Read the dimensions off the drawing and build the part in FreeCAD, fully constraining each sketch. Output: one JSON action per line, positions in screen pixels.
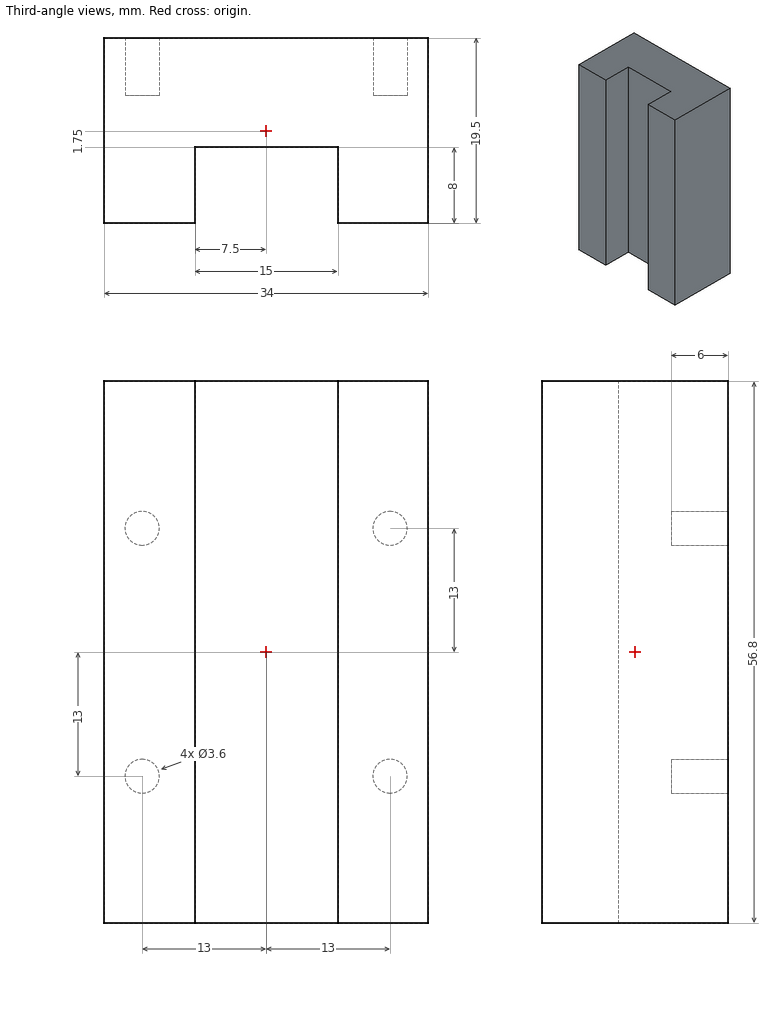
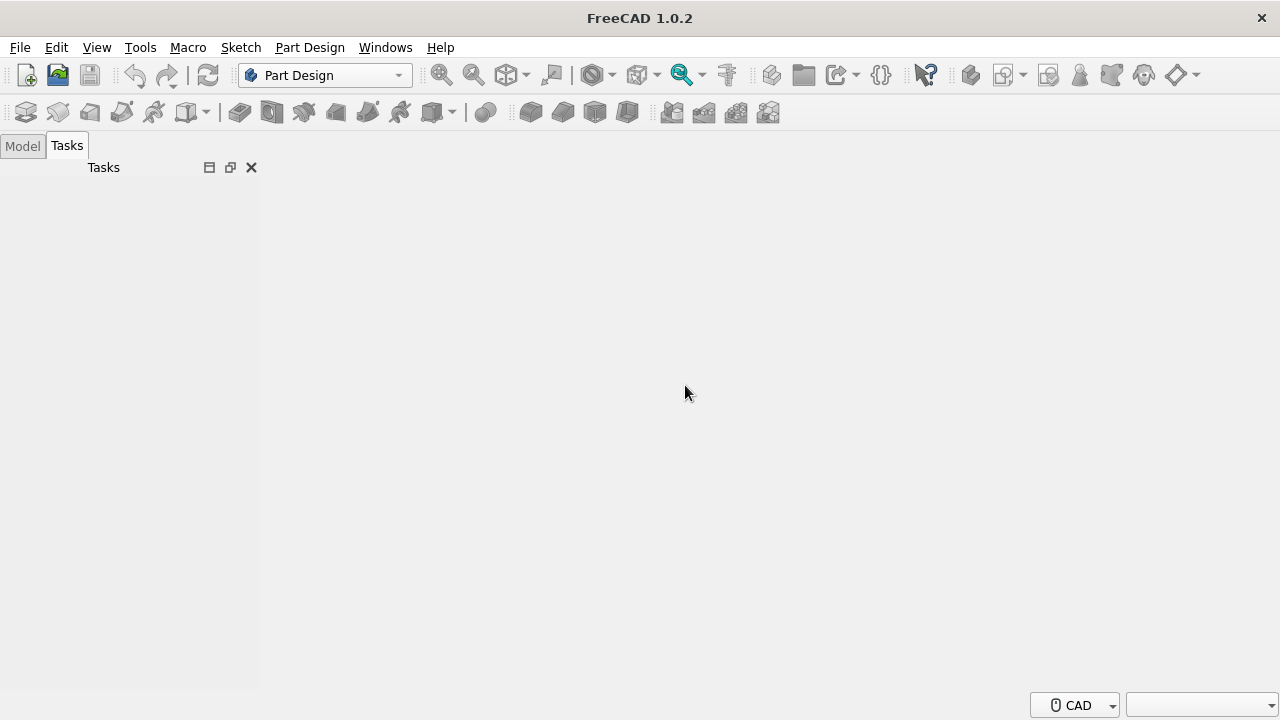
{"action": "left_click", "coordinate": [26, 76]}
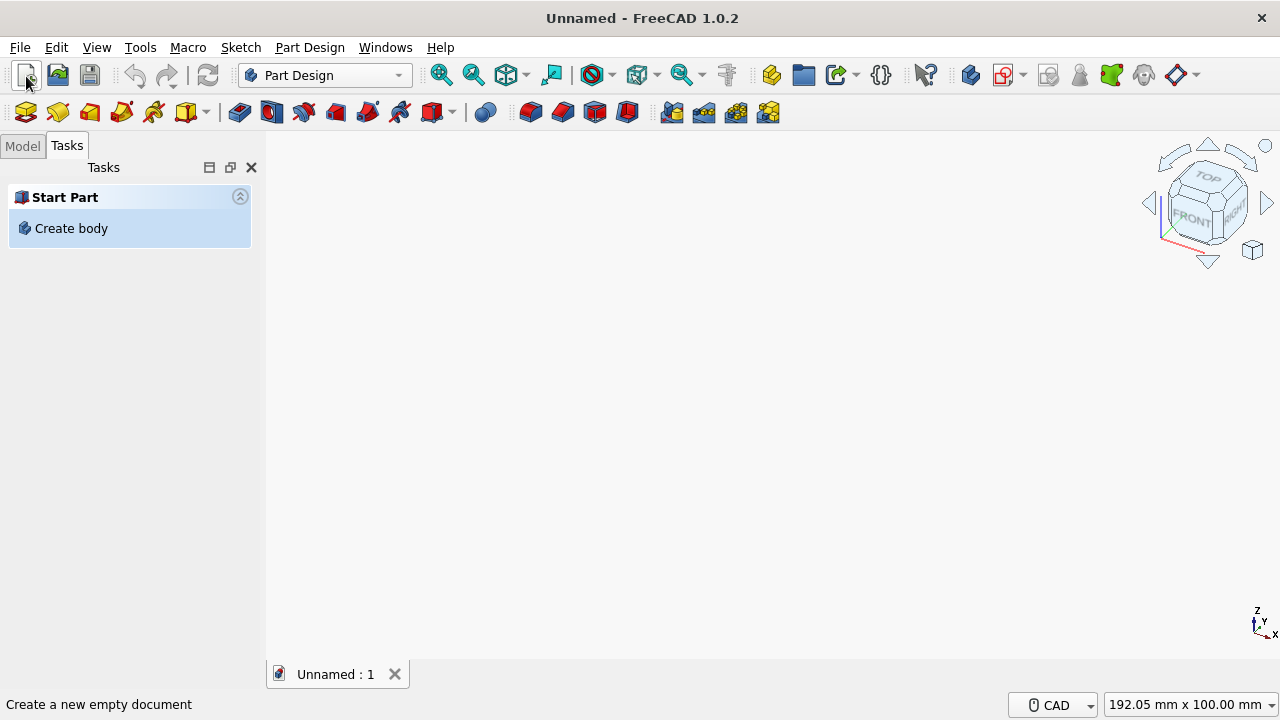
{"action": "left_click", "coordinate": [1004, 76]}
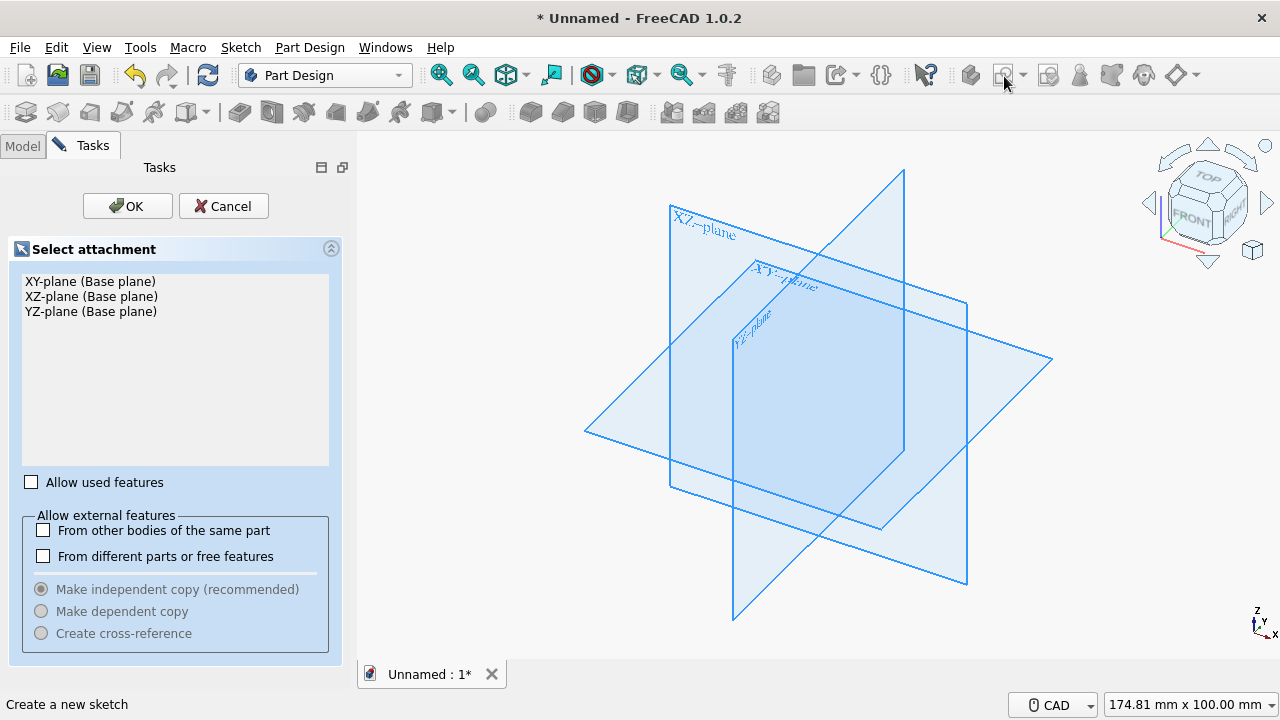
{"action": "left_click", "coordinate": [82, 282]}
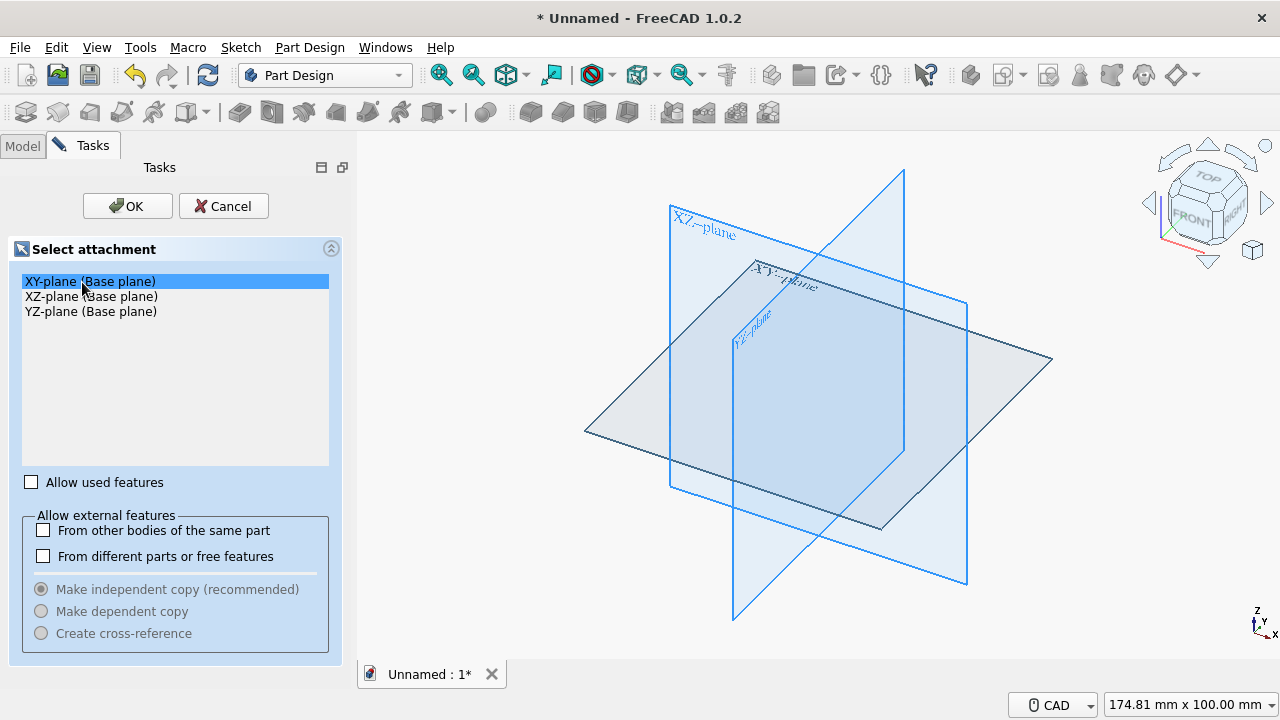
{"action": "left_click", "coordinate": [128, 206]}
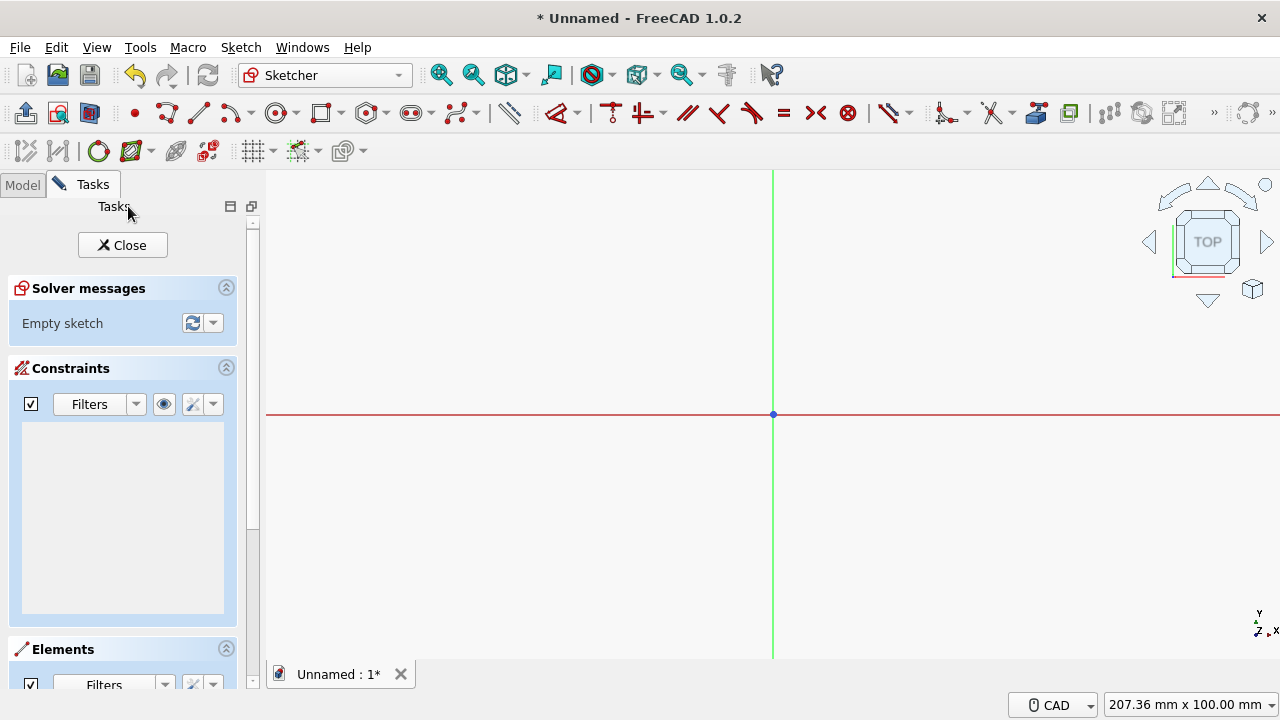
{"action": "scroll", "coordinate": [803, 415], "scroll_direction": "up", "scroll_amount": 6}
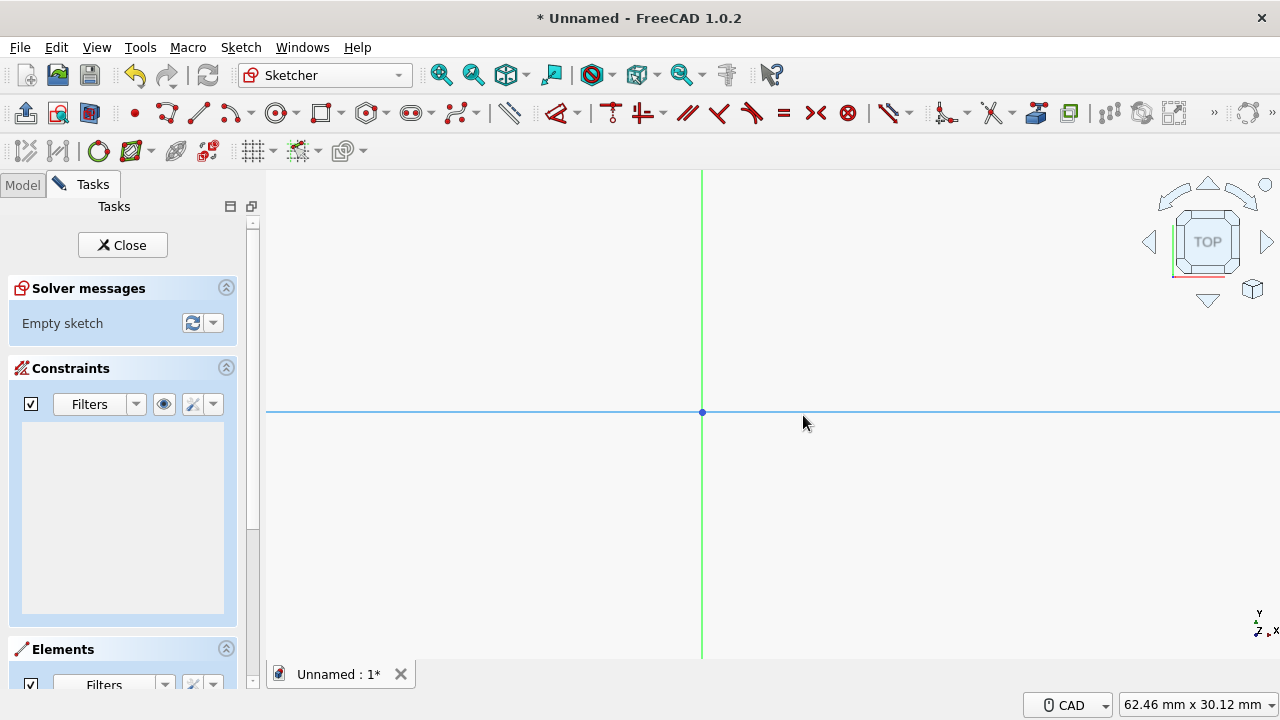
{"action": "left_click", "coordinate": [344, 114]}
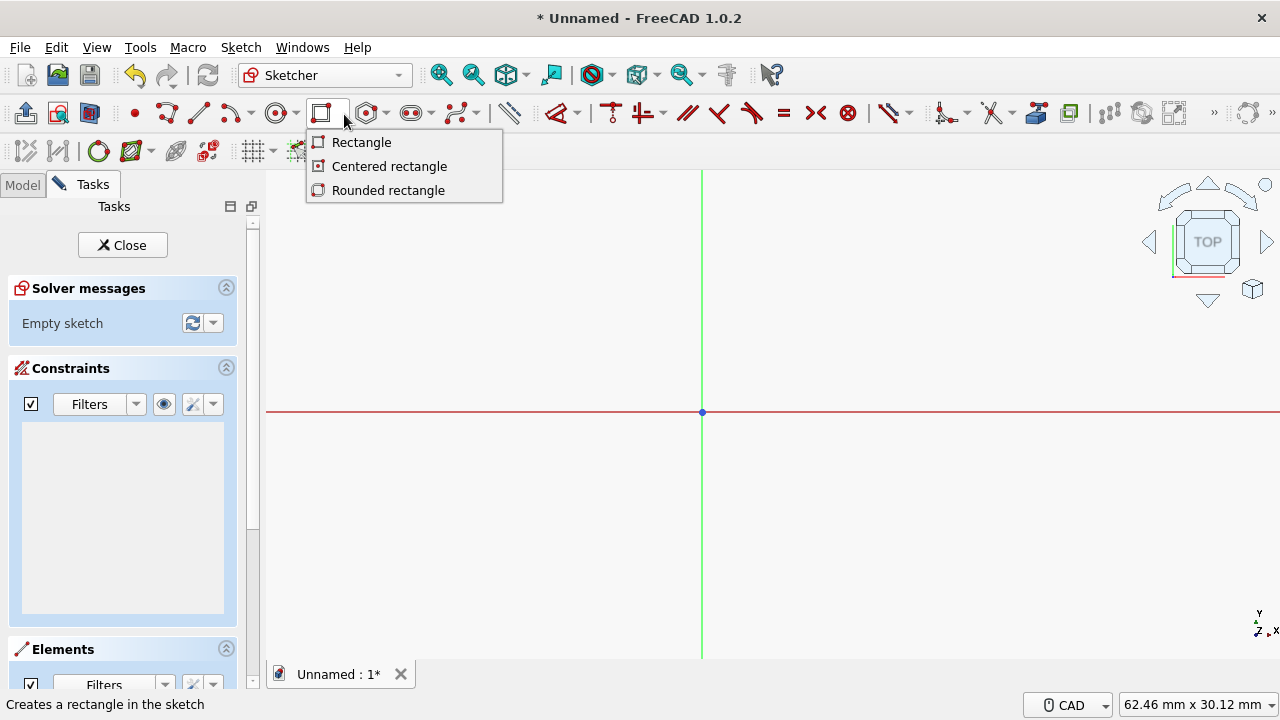
{"action": "left_click", "coordinate": [404, 166]}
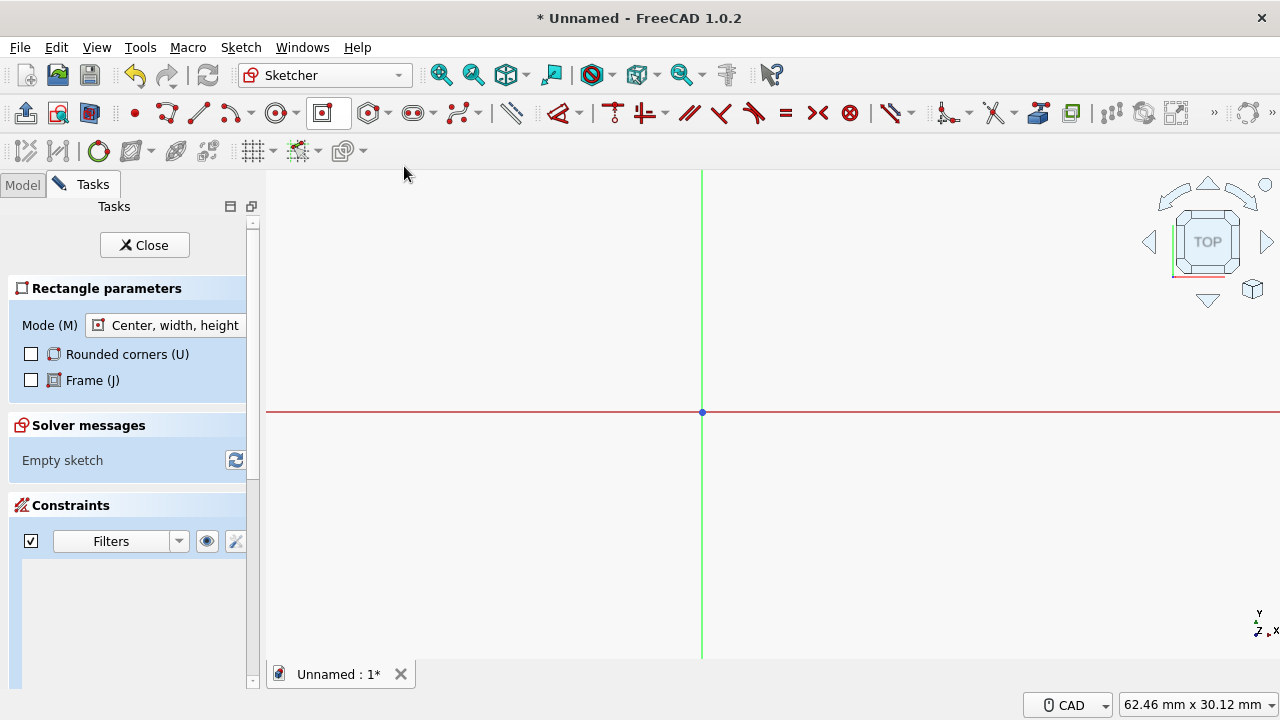
{"action": "left_click", "coordinate": [702, 412]}
{"action": "mouse_move", "coordinate": [978, 254]}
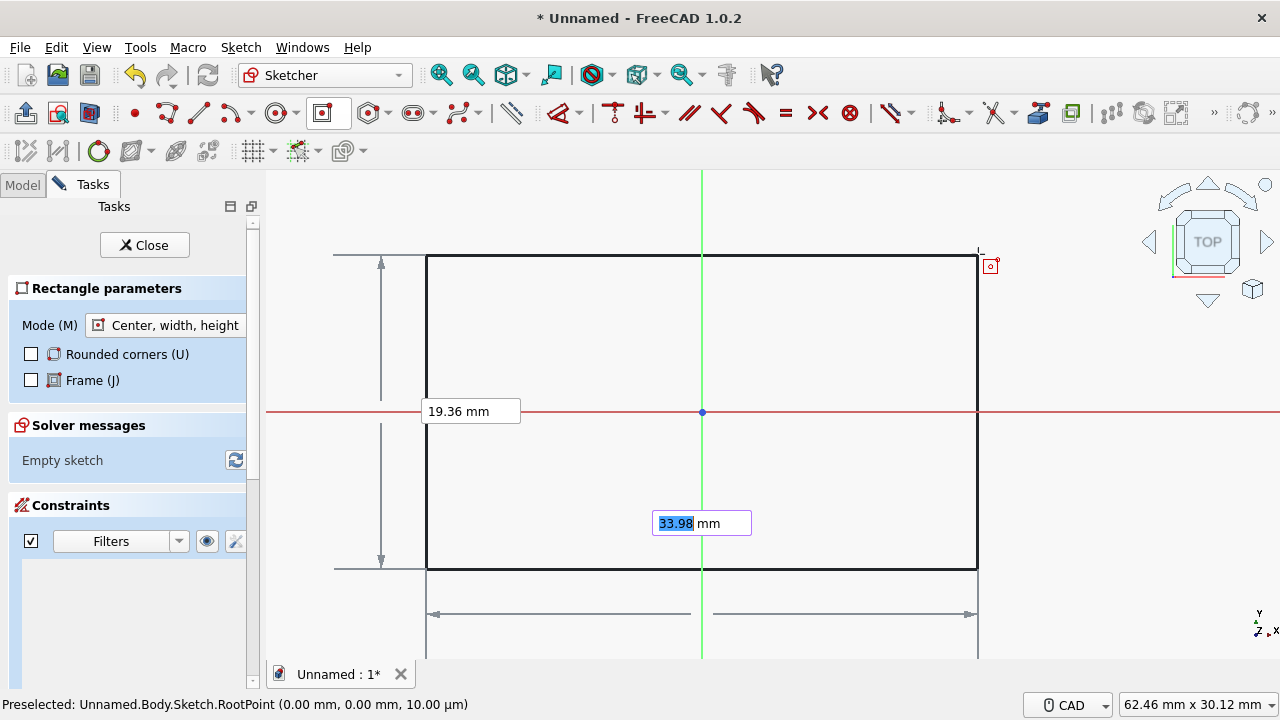
{"action": "type", "text": "34"}
{"action": "key", "text": "Tab"}
{"action": "type", "text": "19.5"}
{"action": "key", "text": "Return"}
{"action": "key", "text": "Escape"}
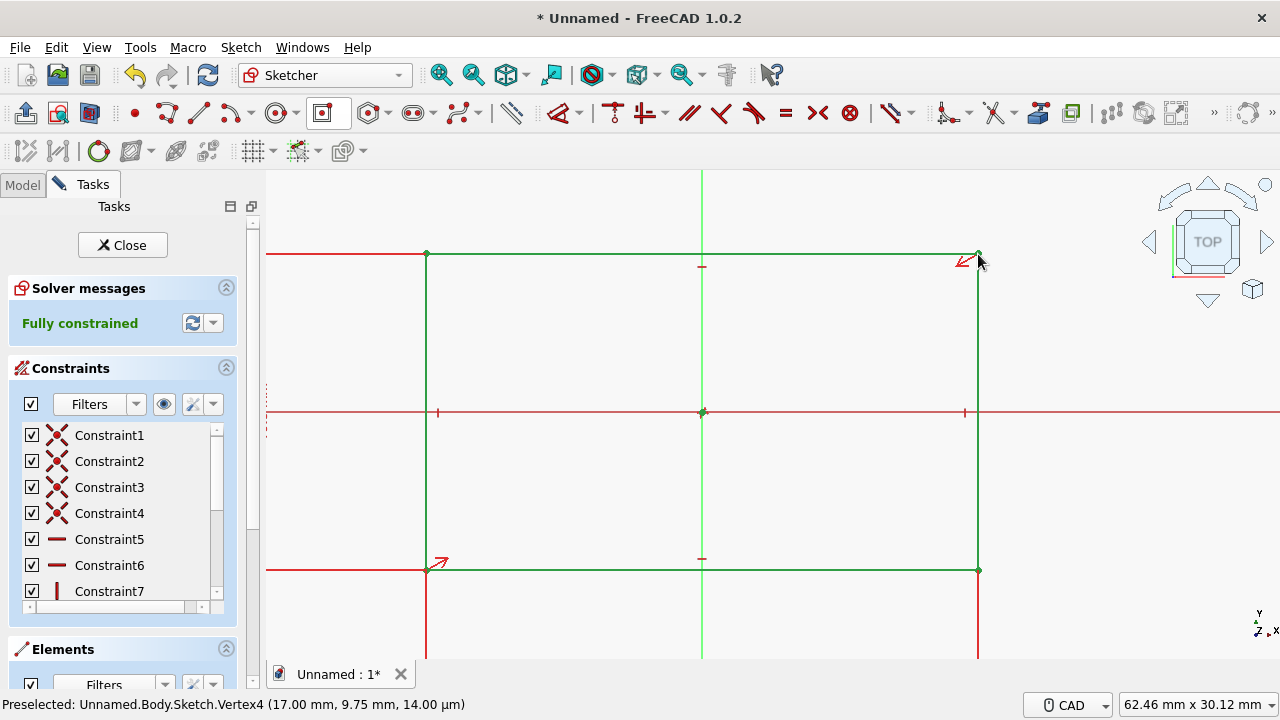
{"action": "left_click", "coordinate": [123, 245]}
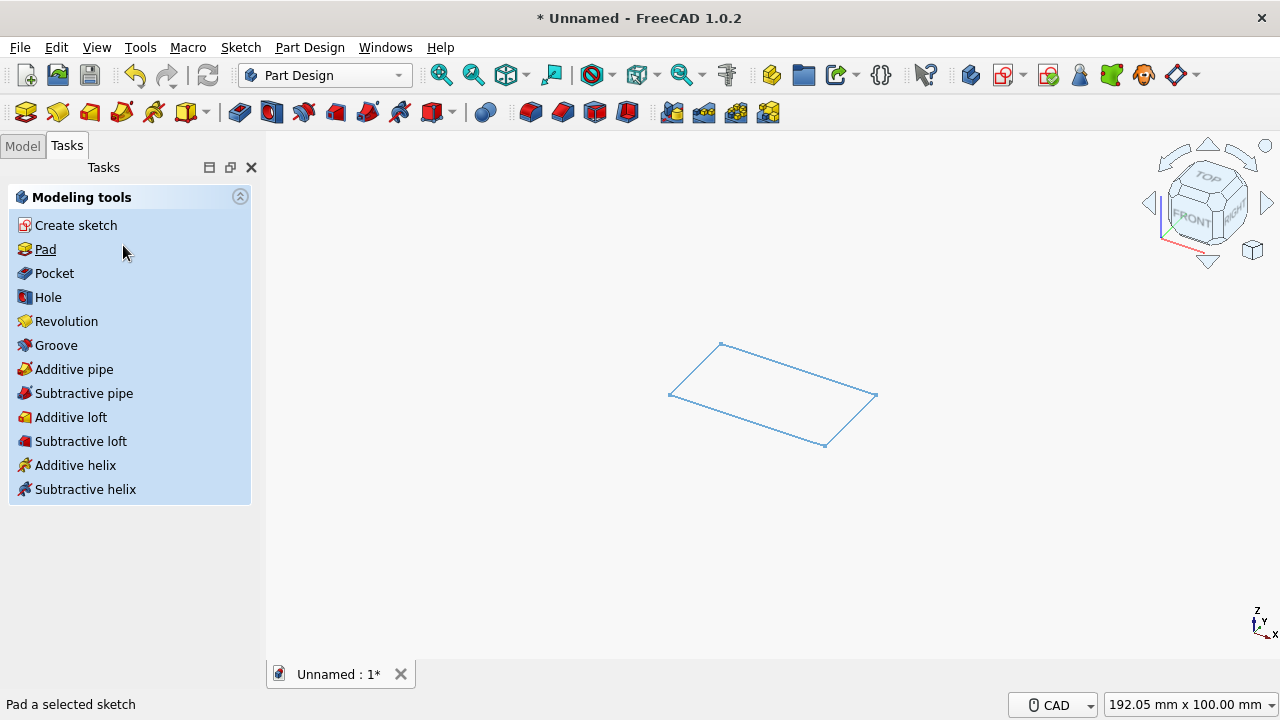
{"action": "left_click", "coordinate": [26, 112]}